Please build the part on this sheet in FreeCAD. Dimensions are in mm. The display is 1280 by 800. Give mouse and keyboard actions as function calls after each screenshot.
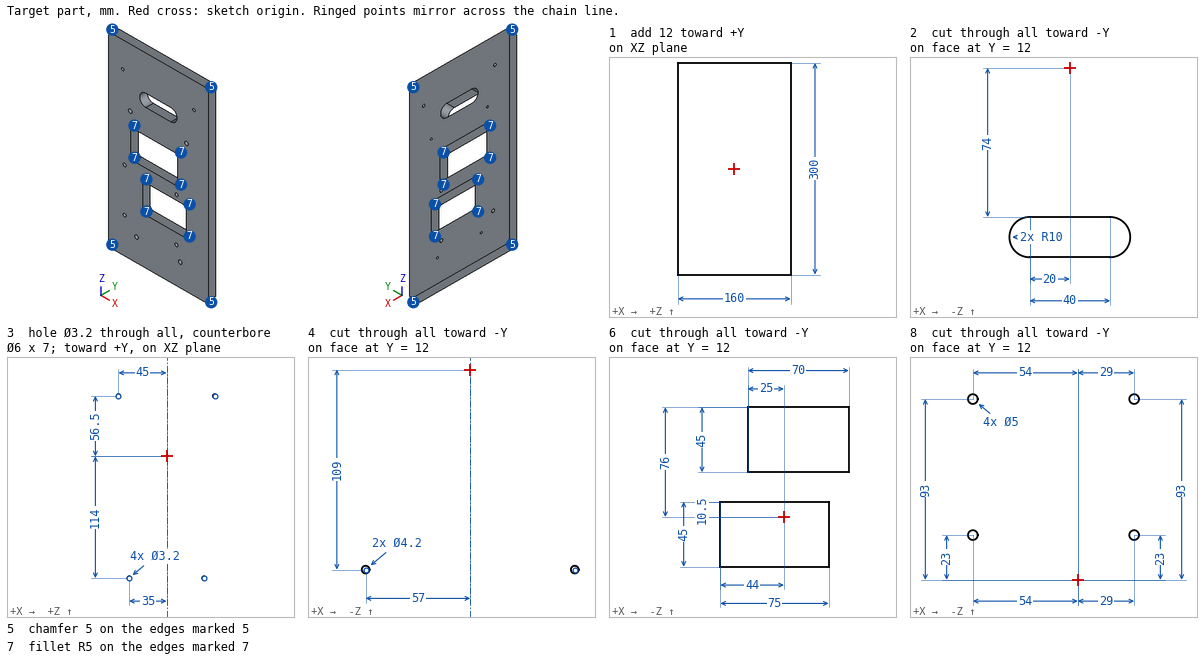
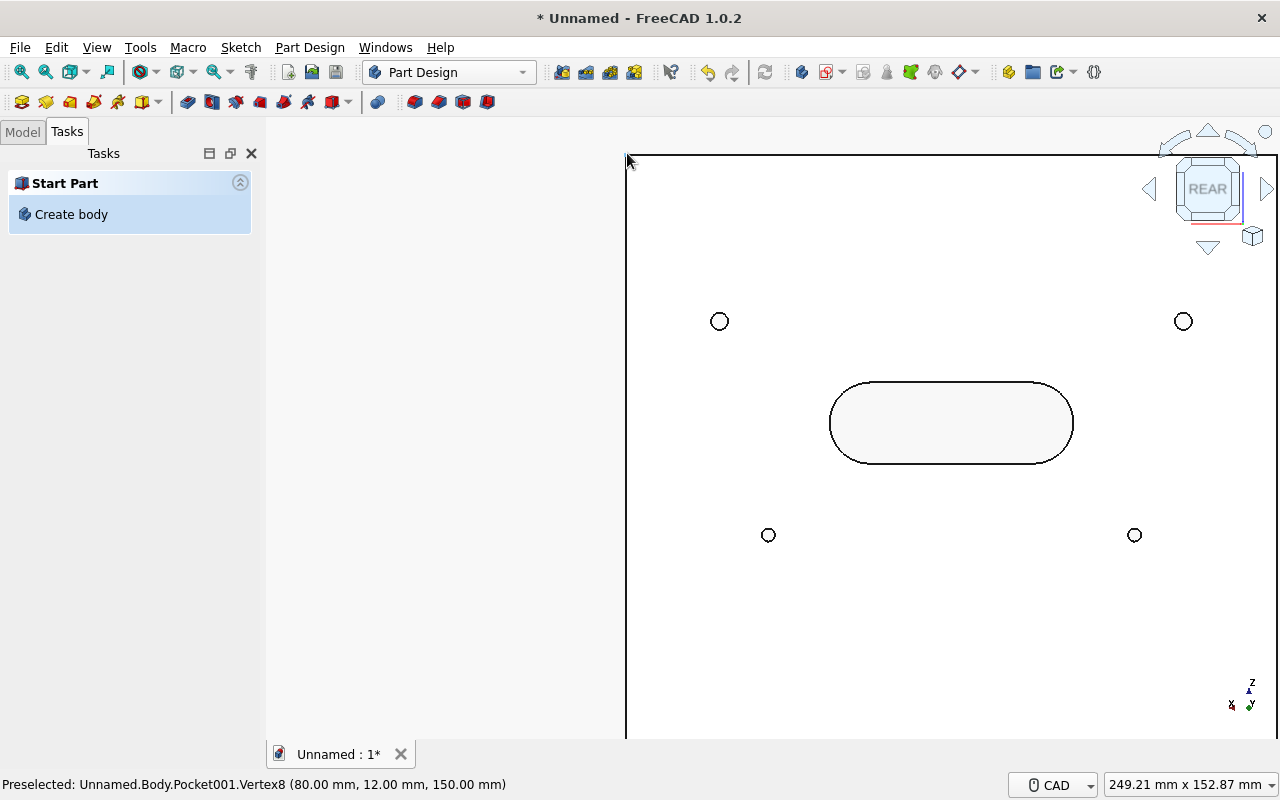
click(22, 72)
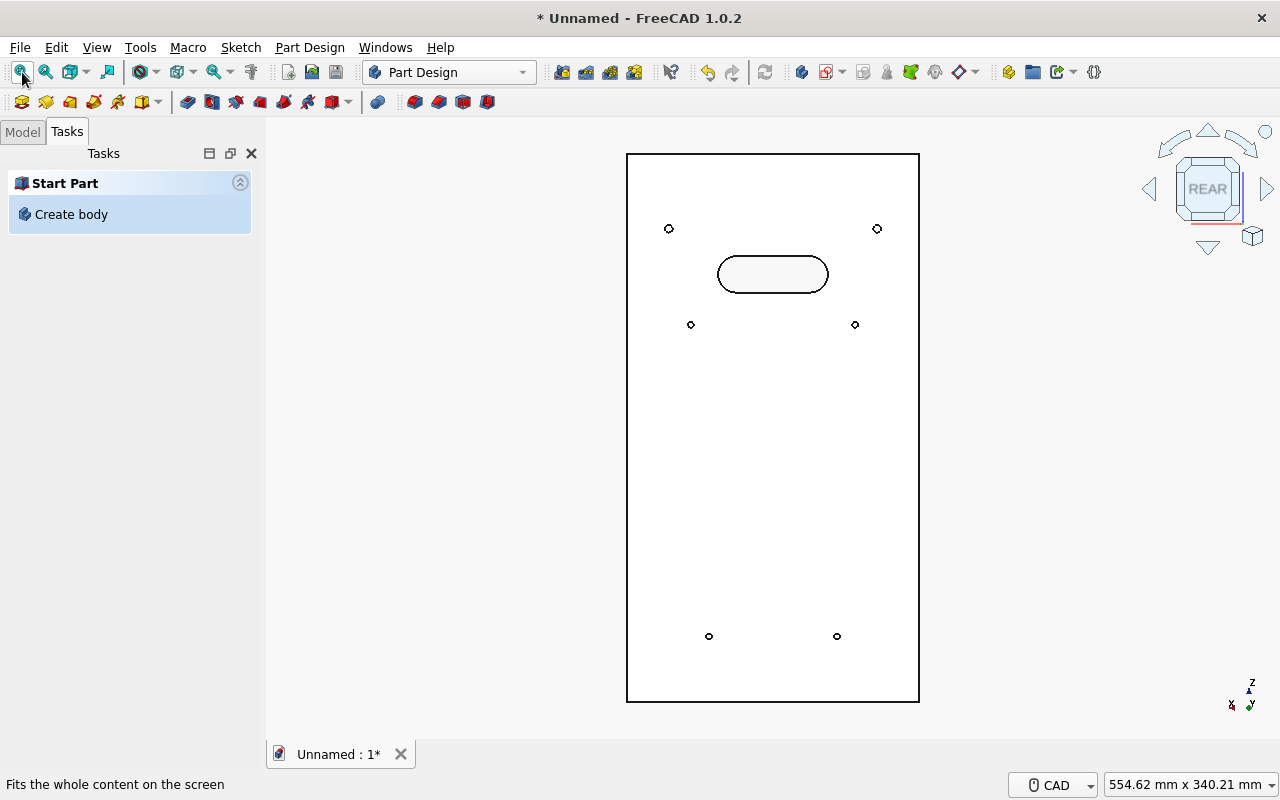
key(0)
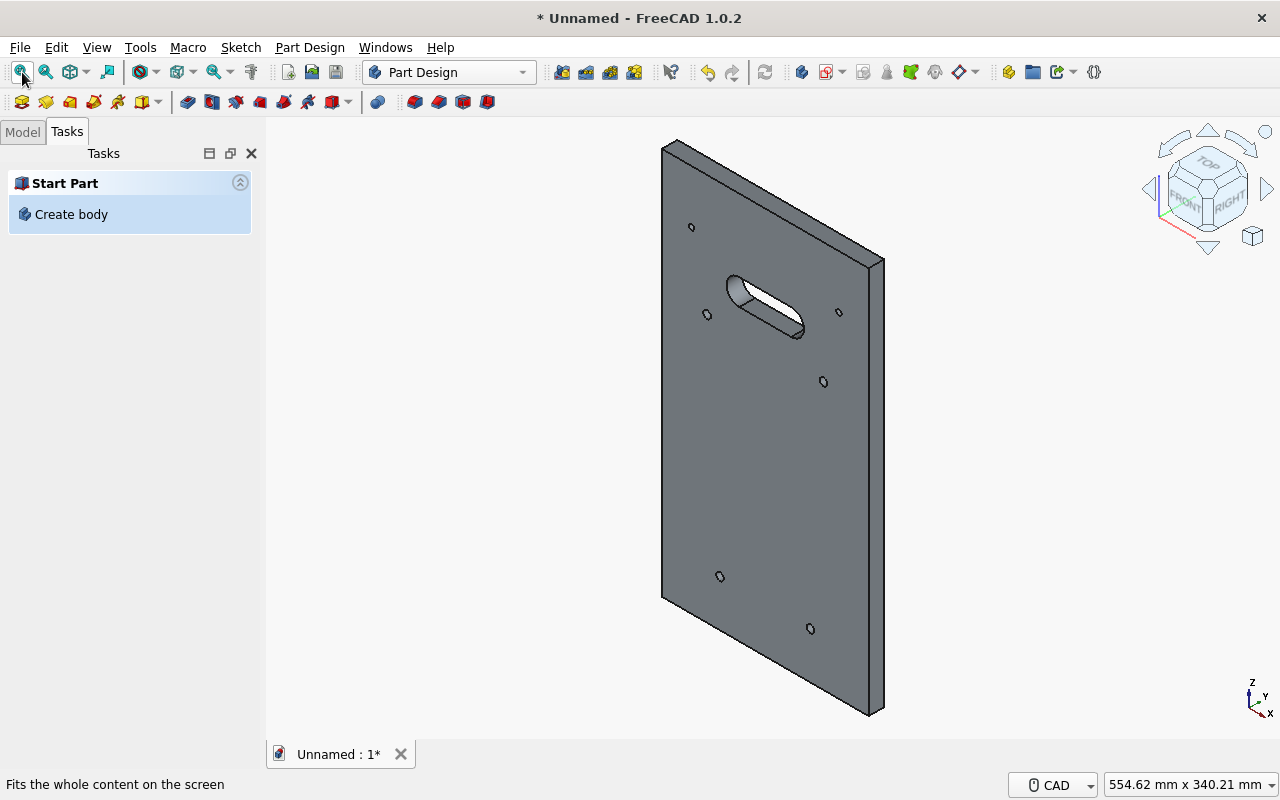
click(876, 263)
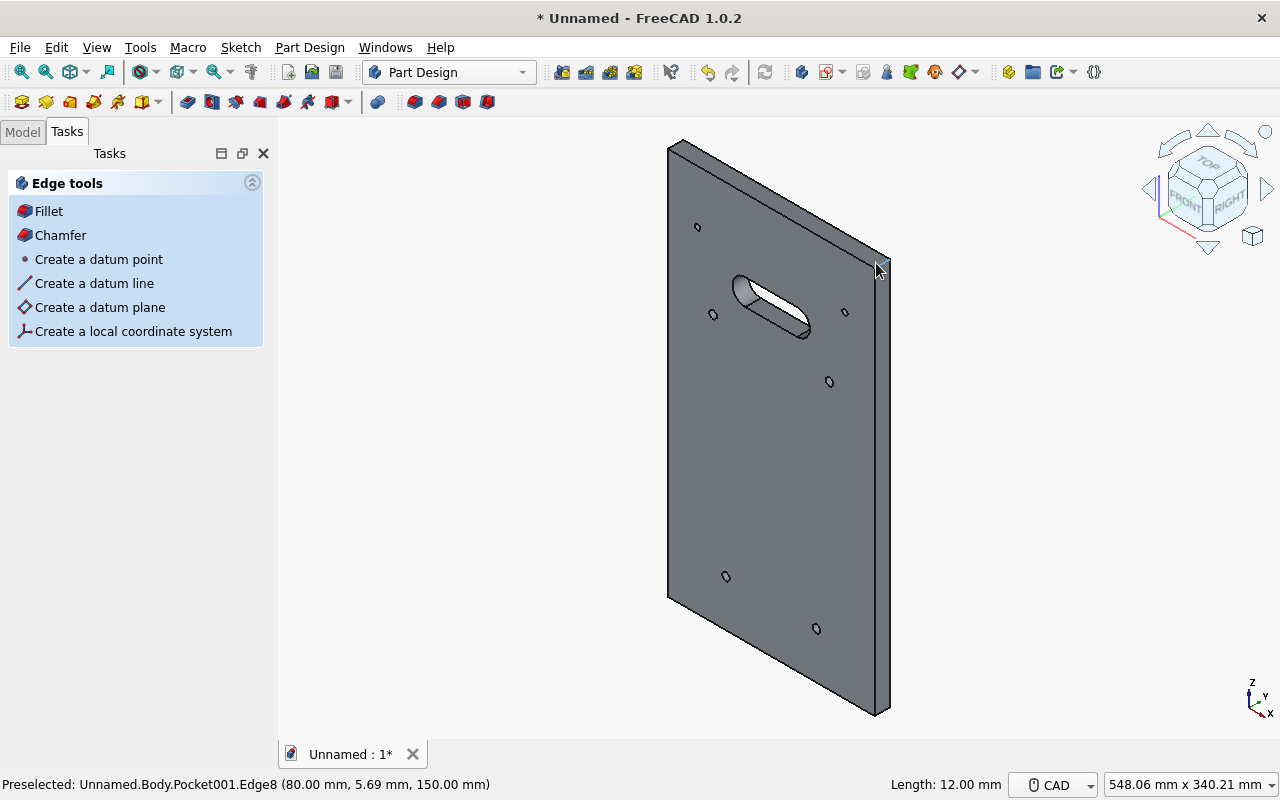
key(2)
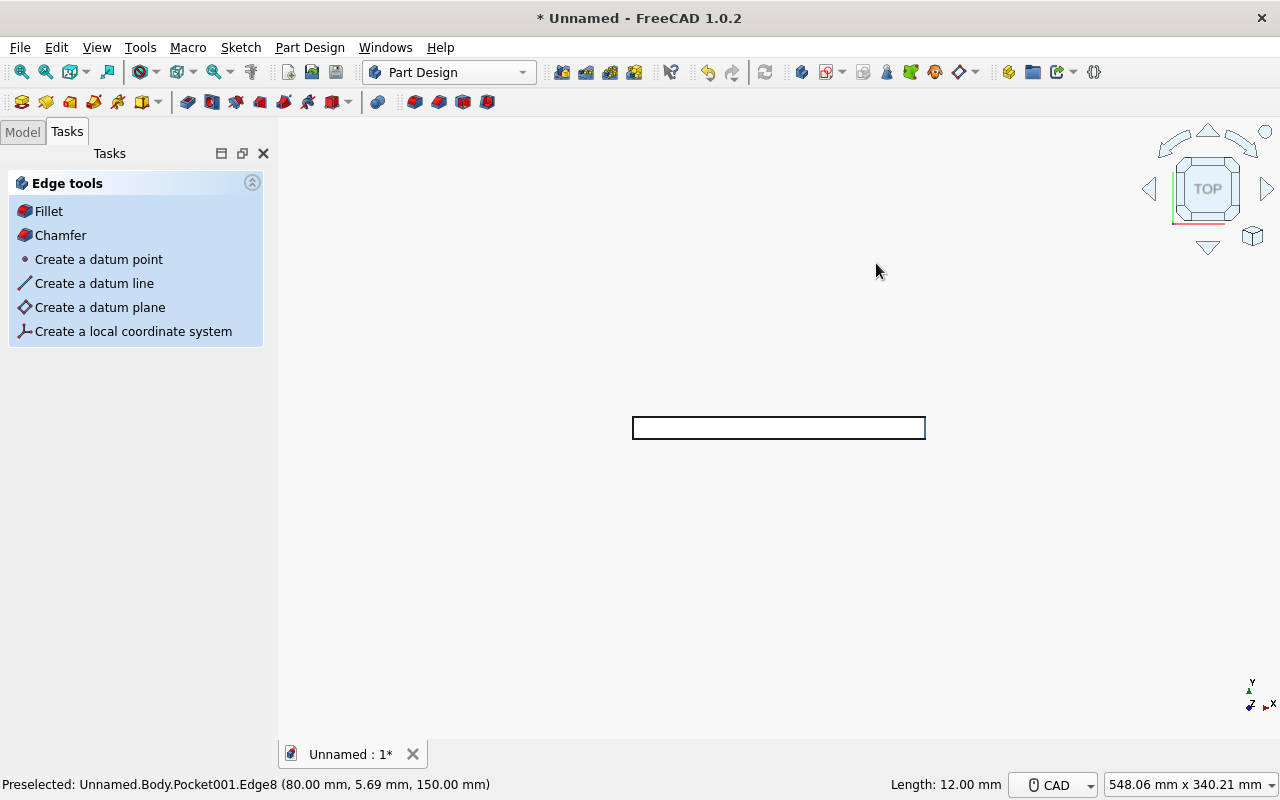
click(22, 72)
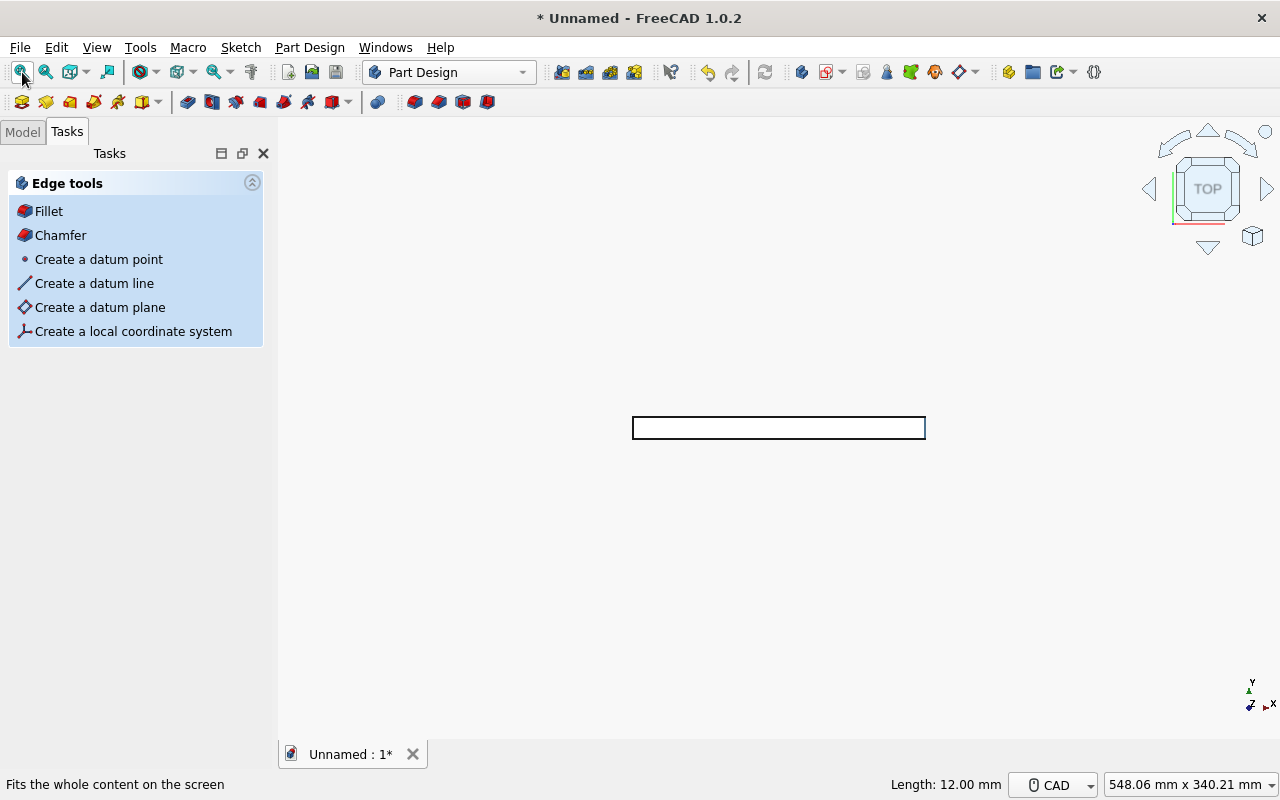
click(633, 427, ctrl)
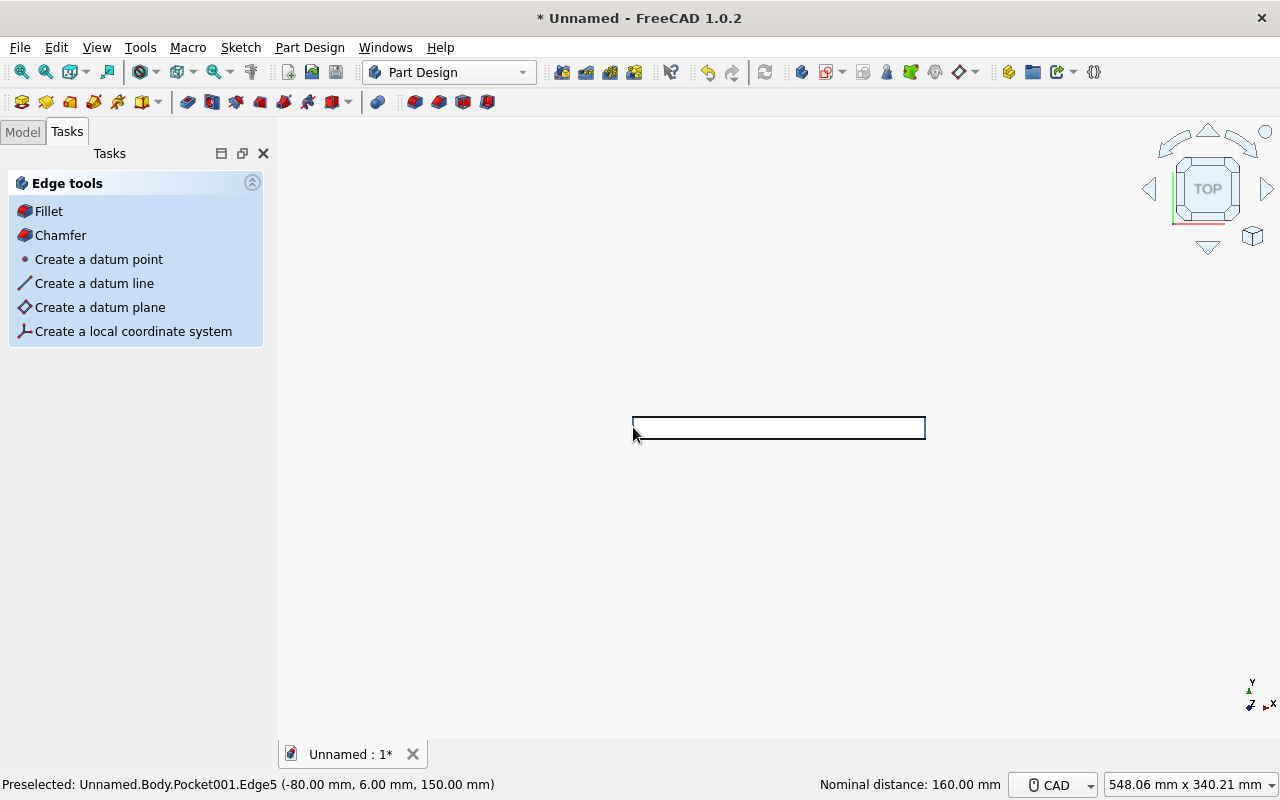
scroll(633, 427, up, 4)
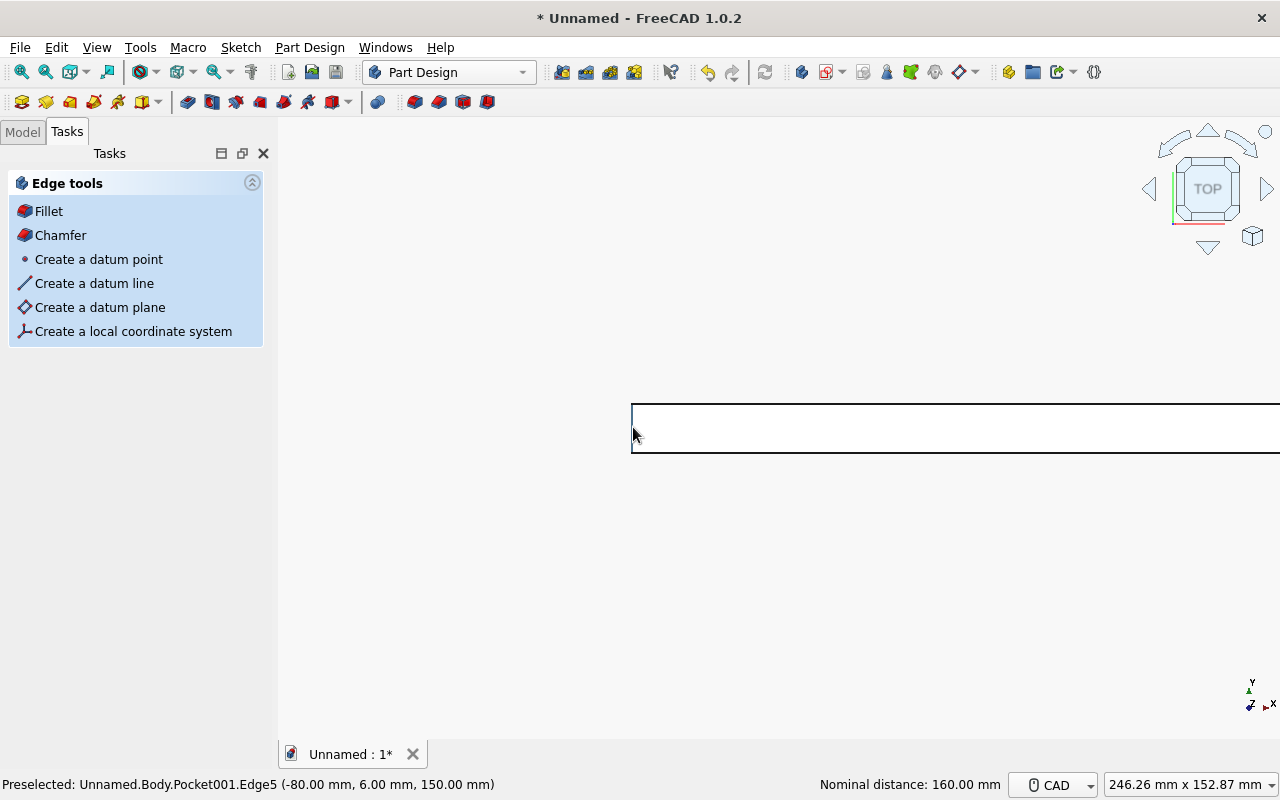
click(22, 72)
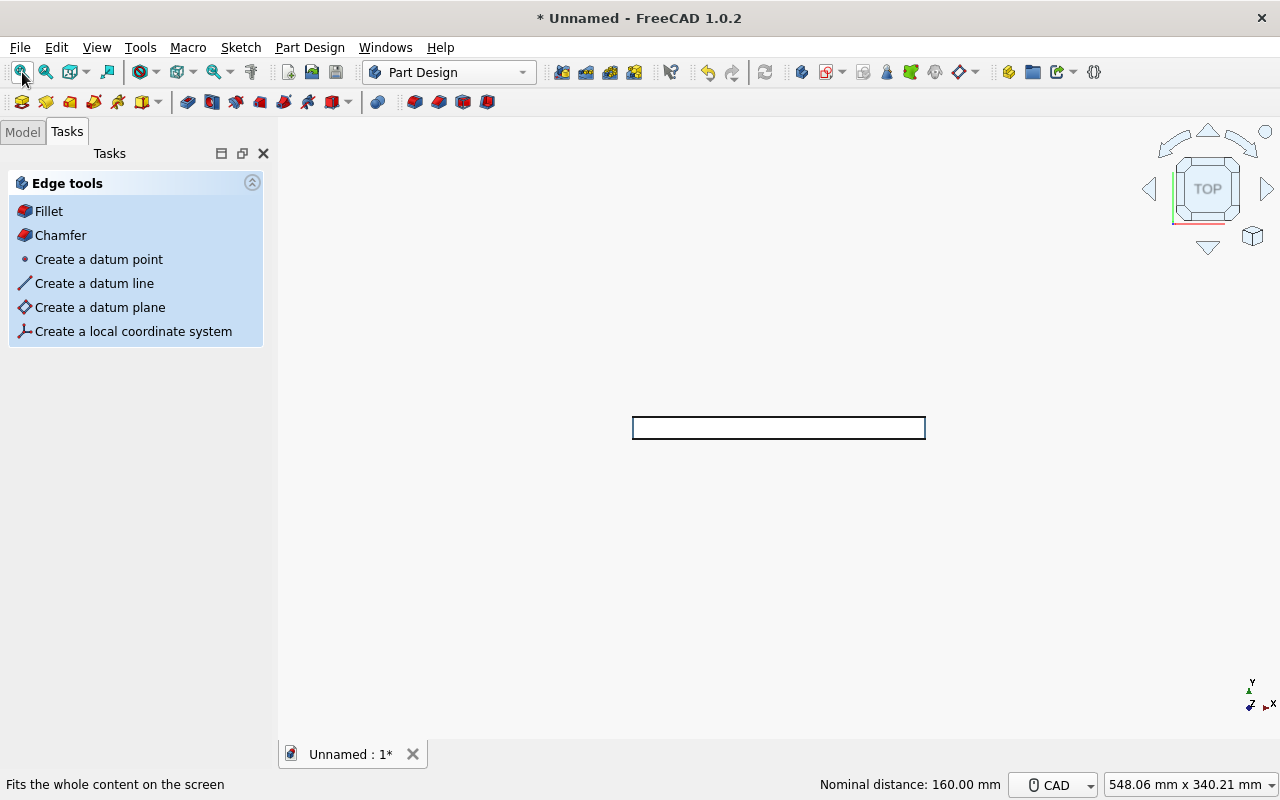
key(1)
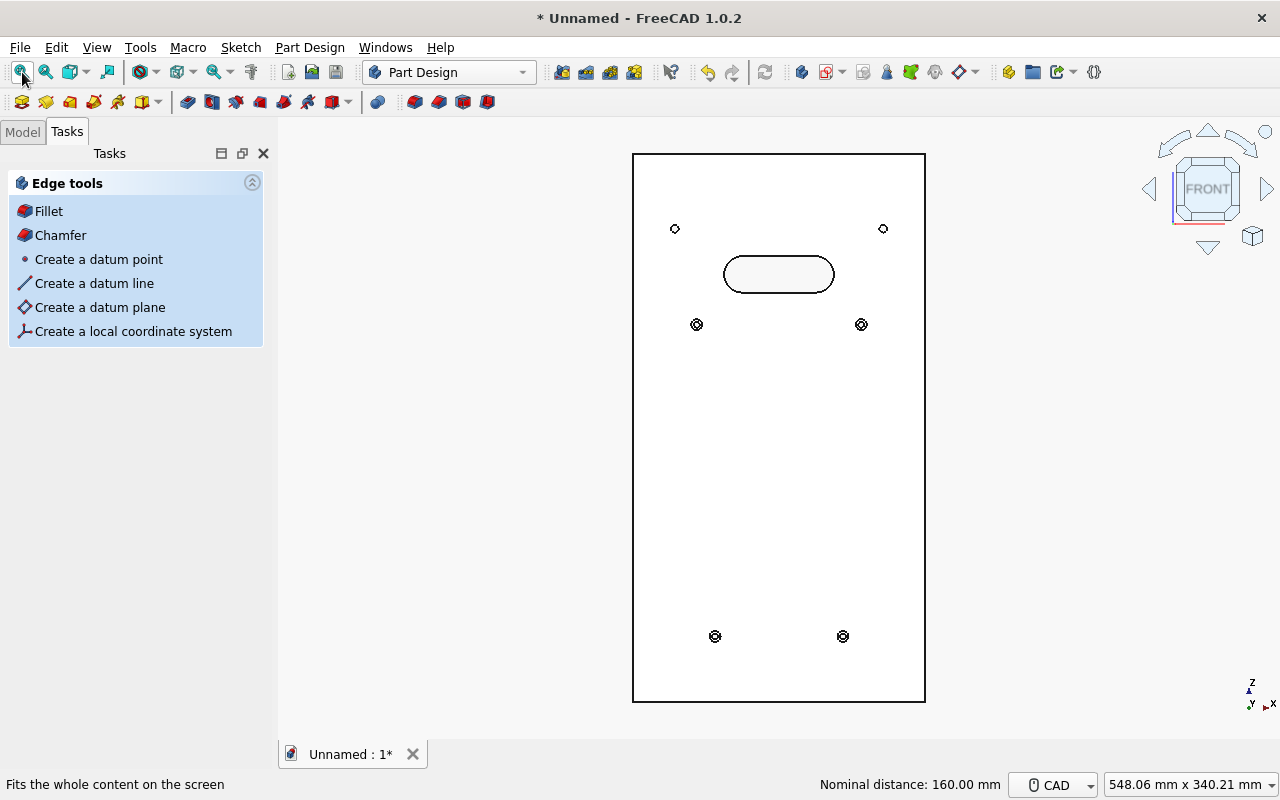
scroll(633, 701, up, 4)